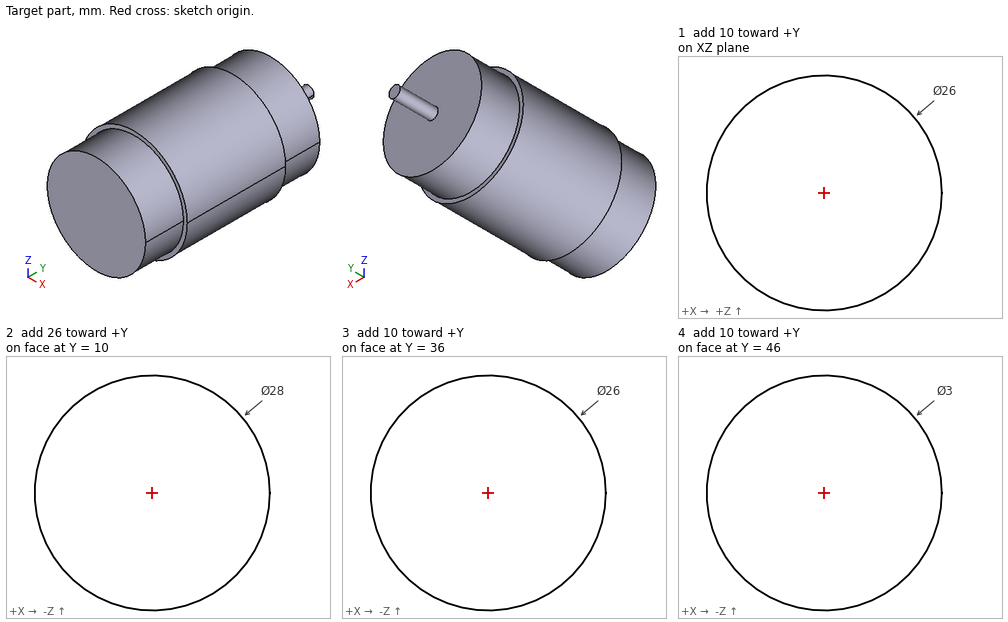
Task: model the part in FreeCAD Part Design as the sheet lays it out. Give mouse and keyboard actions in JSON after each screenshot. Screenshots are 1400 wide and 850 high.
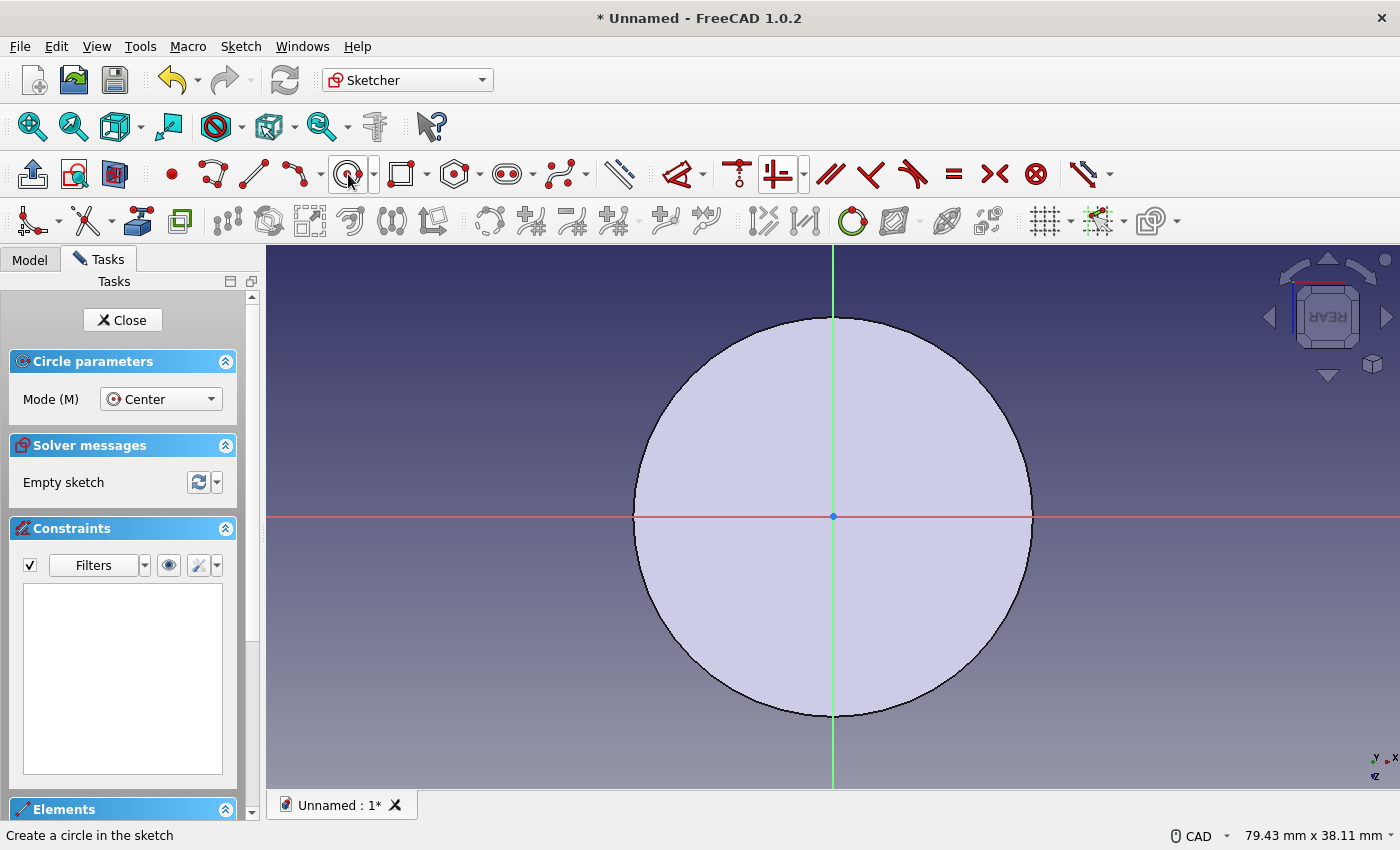
{"action": "left_click", "coordinate": [833, 517]}
{"action": "mouse_move", "coordinate": [964, 386]}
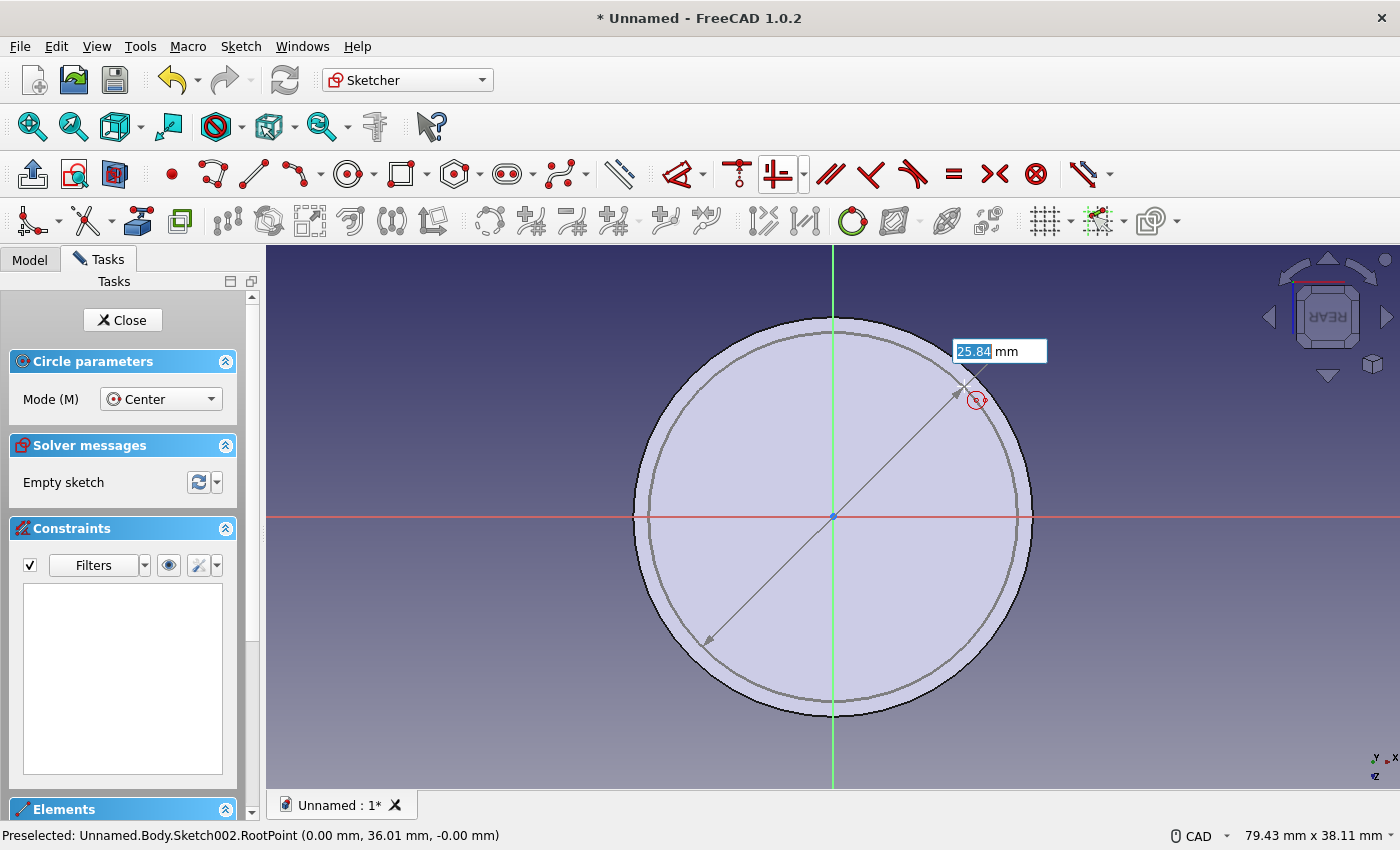
{"action": "type", "text": "26"}
{"action": "key", "text": "Return"}
{"action": "key", "text": "Escape"}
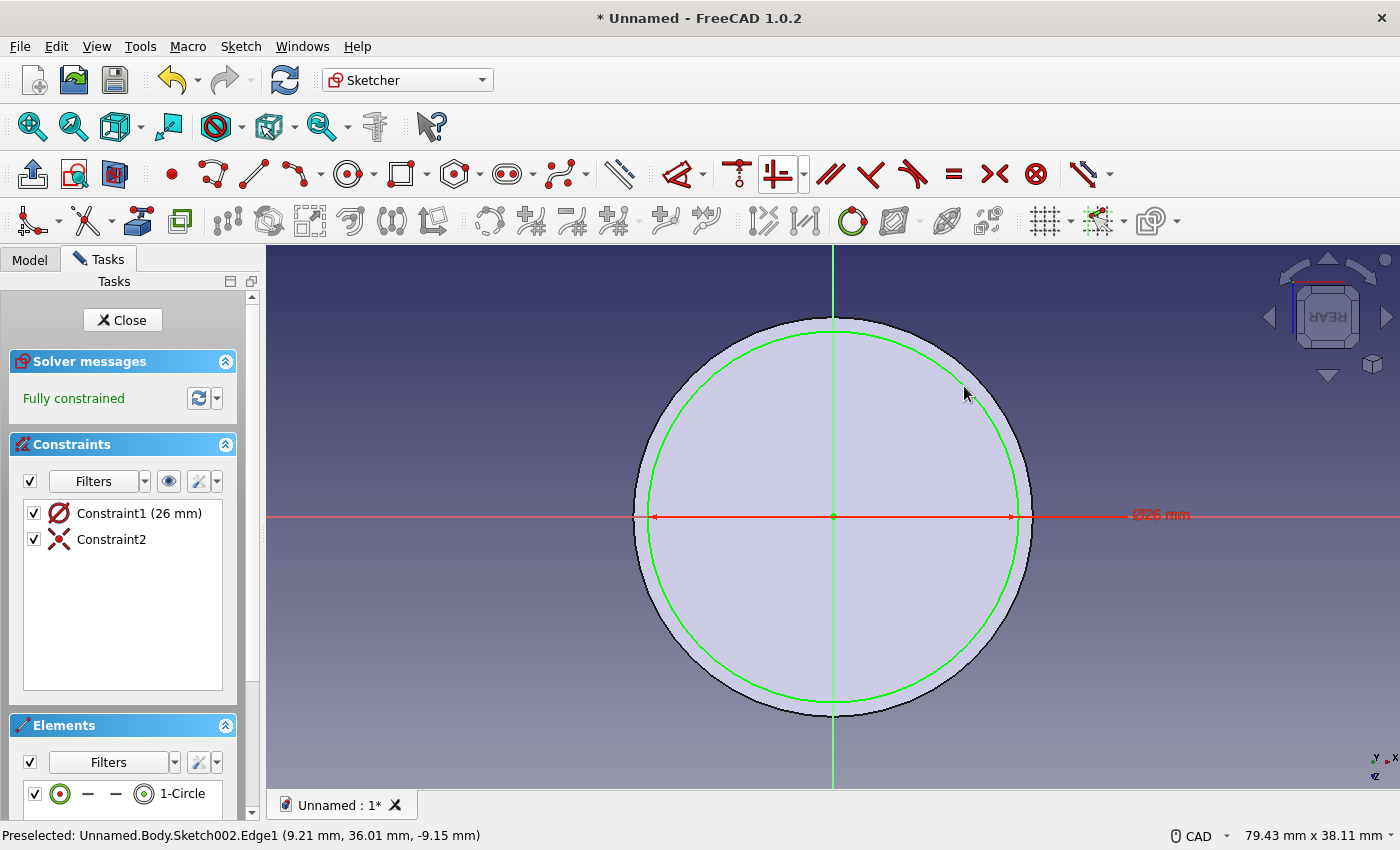
{"action": "left_click", "coordinate": [123, 320]}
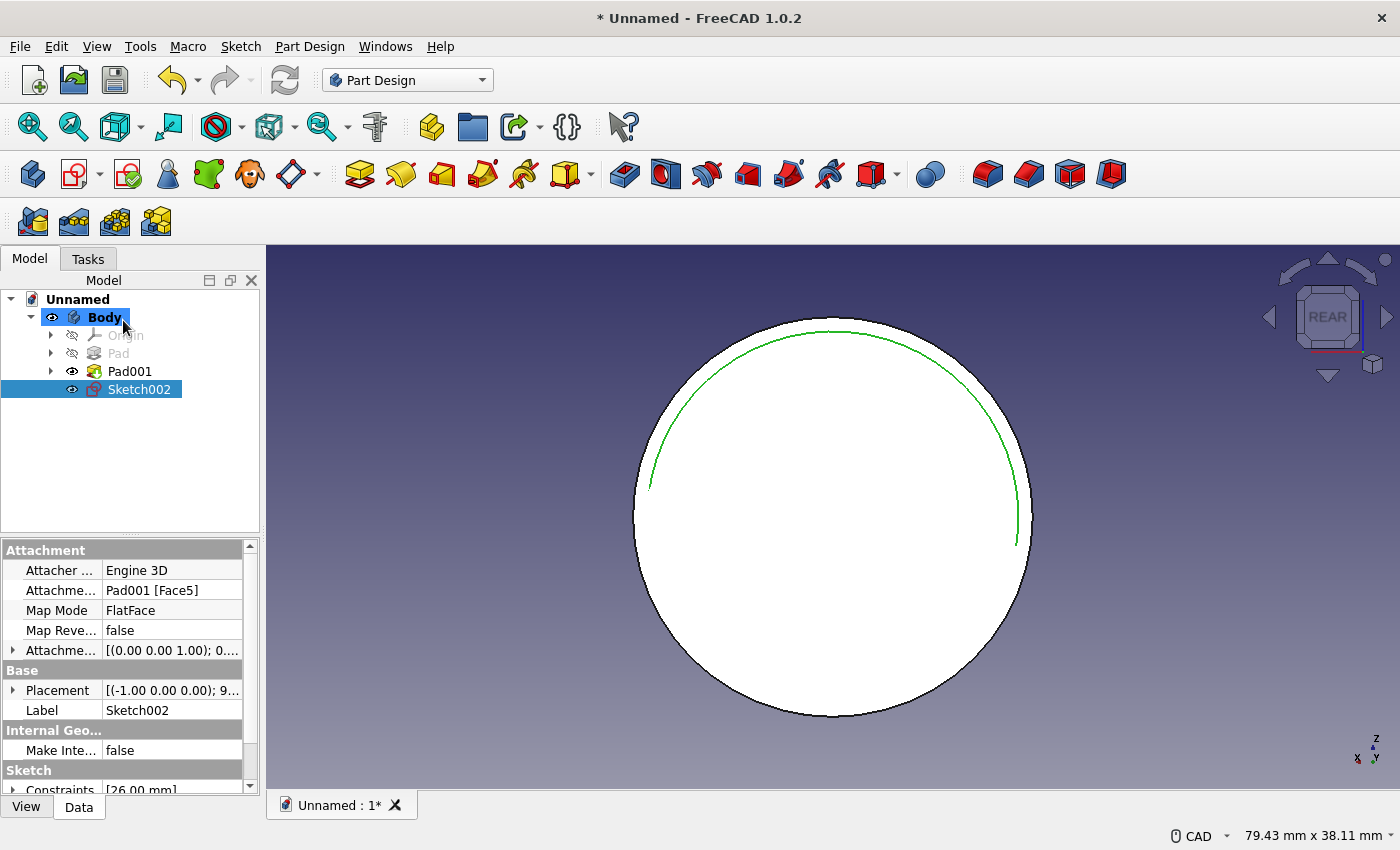
{"action": "left_click", "coordinate": [360, 174]}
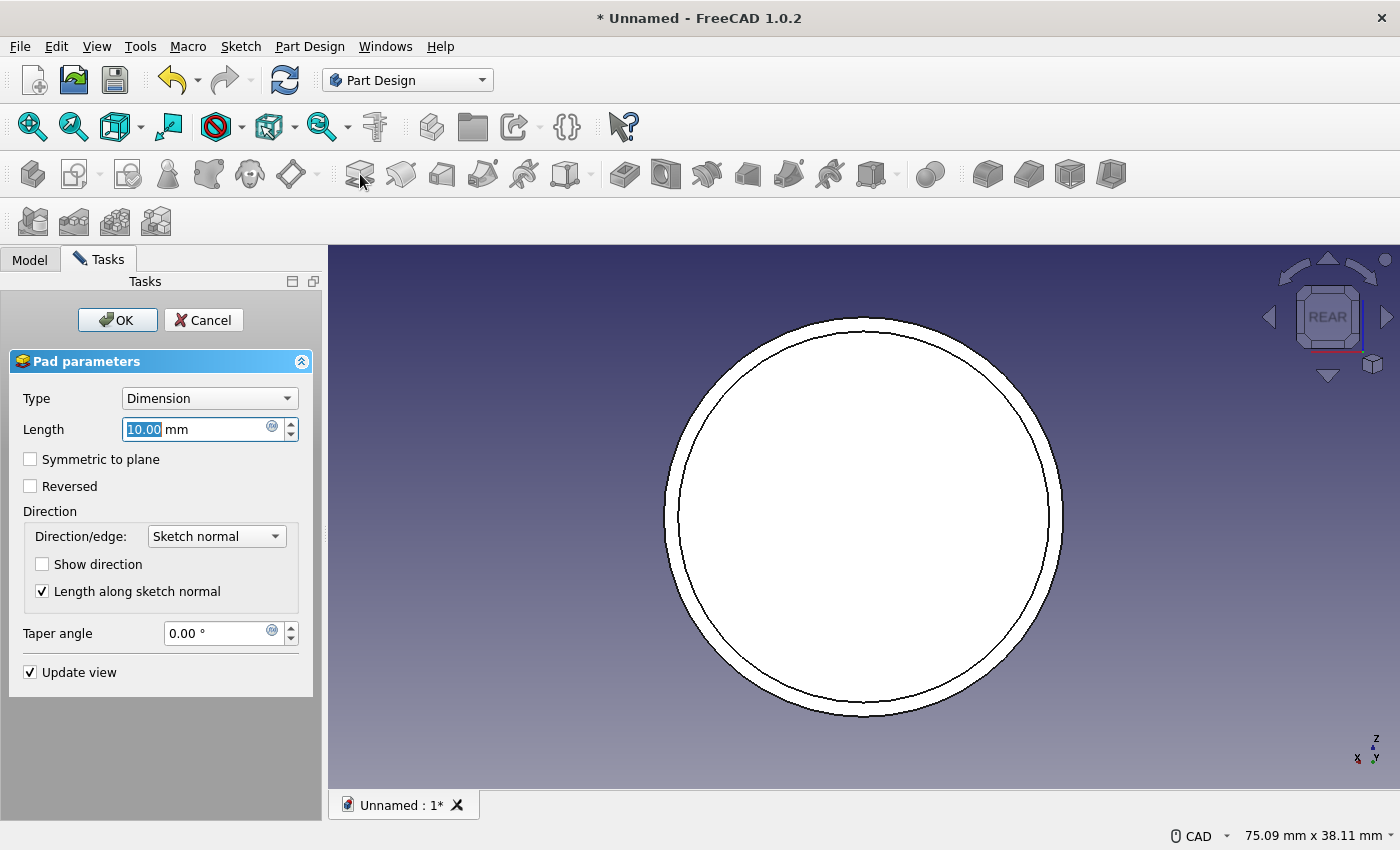
{"action": "type", "text": "10"}
{"action": "key", "text": "Tab"}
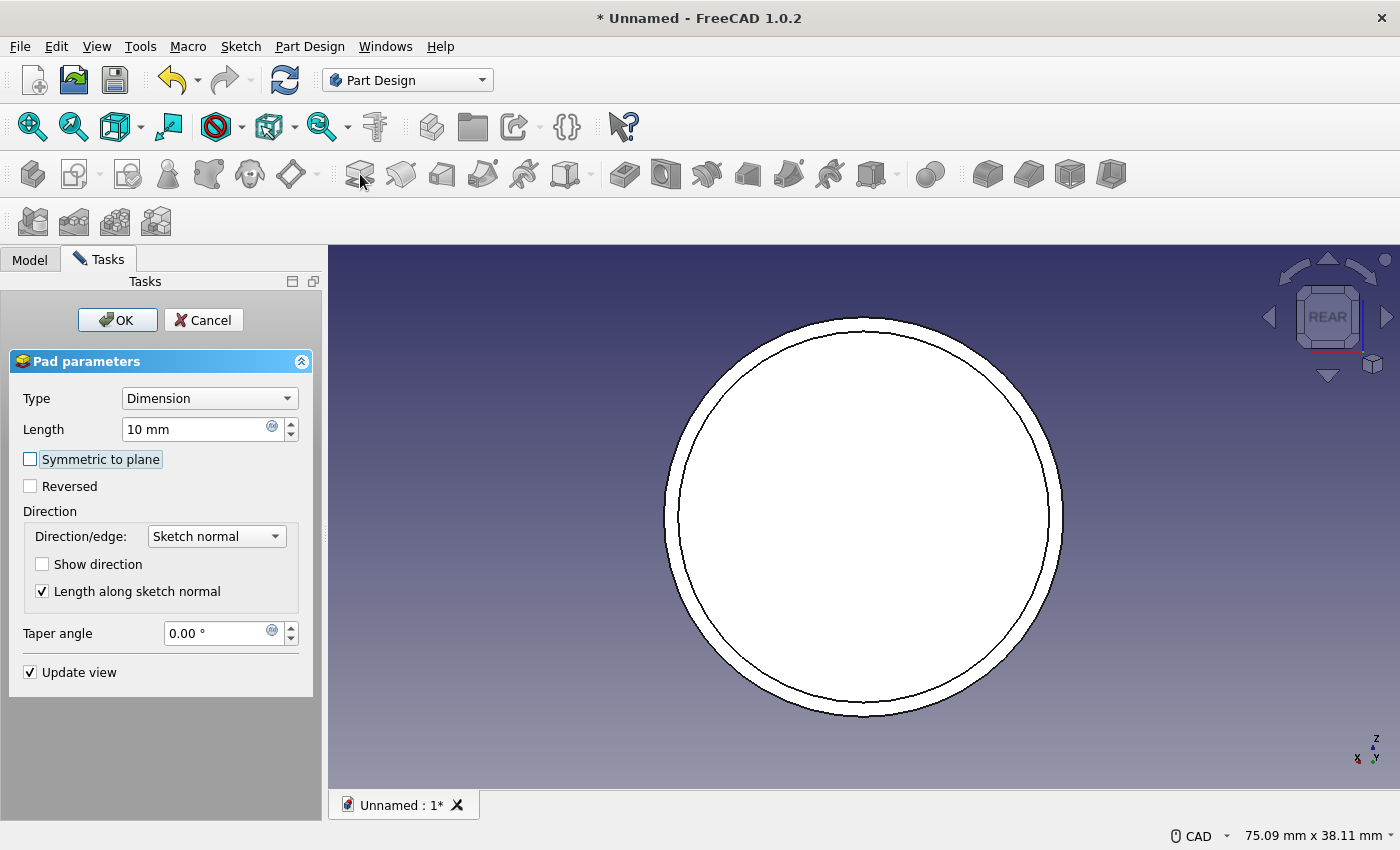
{"action": "left_click", "coordinate": [118, 320]}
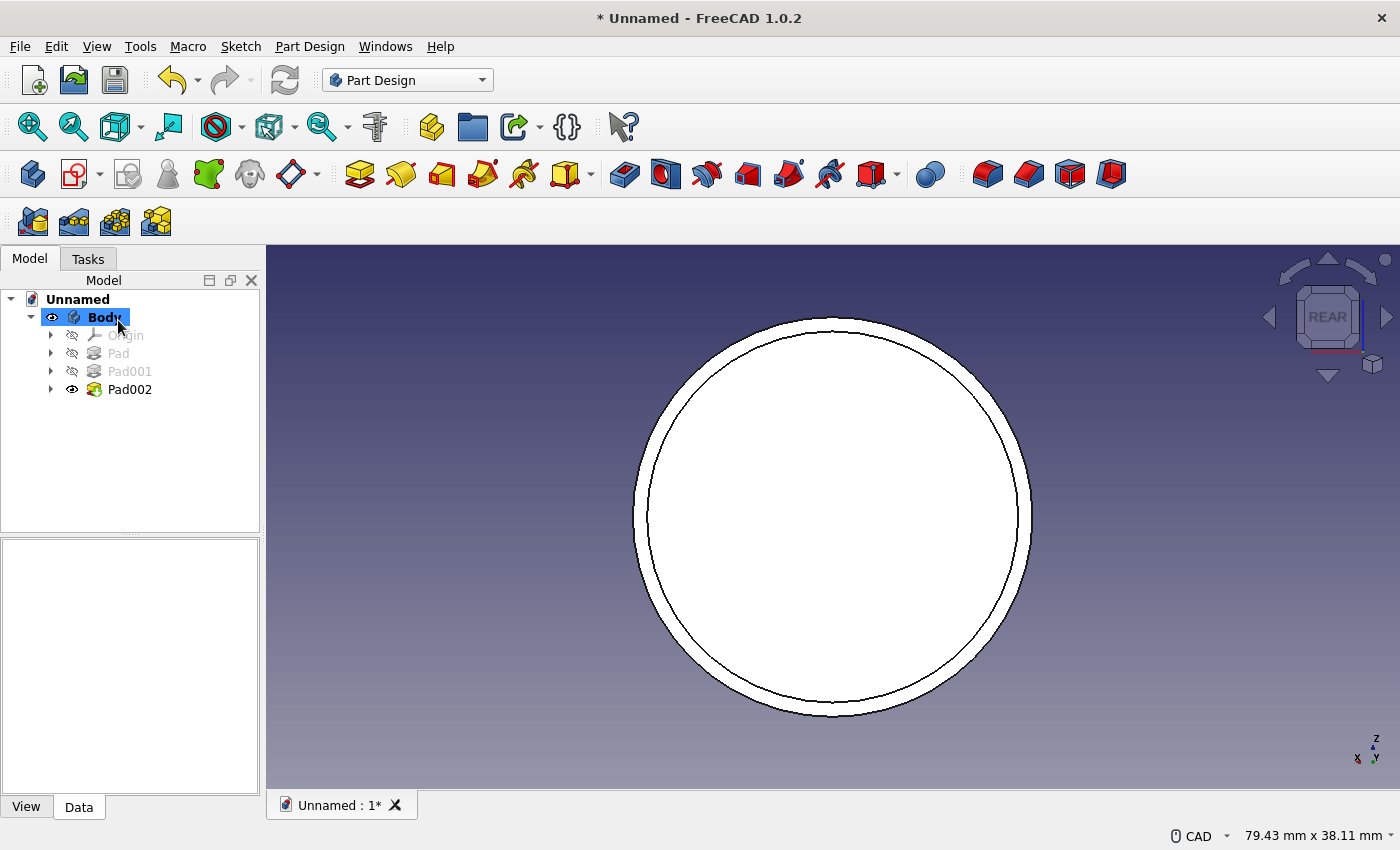
{"action": "left_click", "coordinate": [833, 516]}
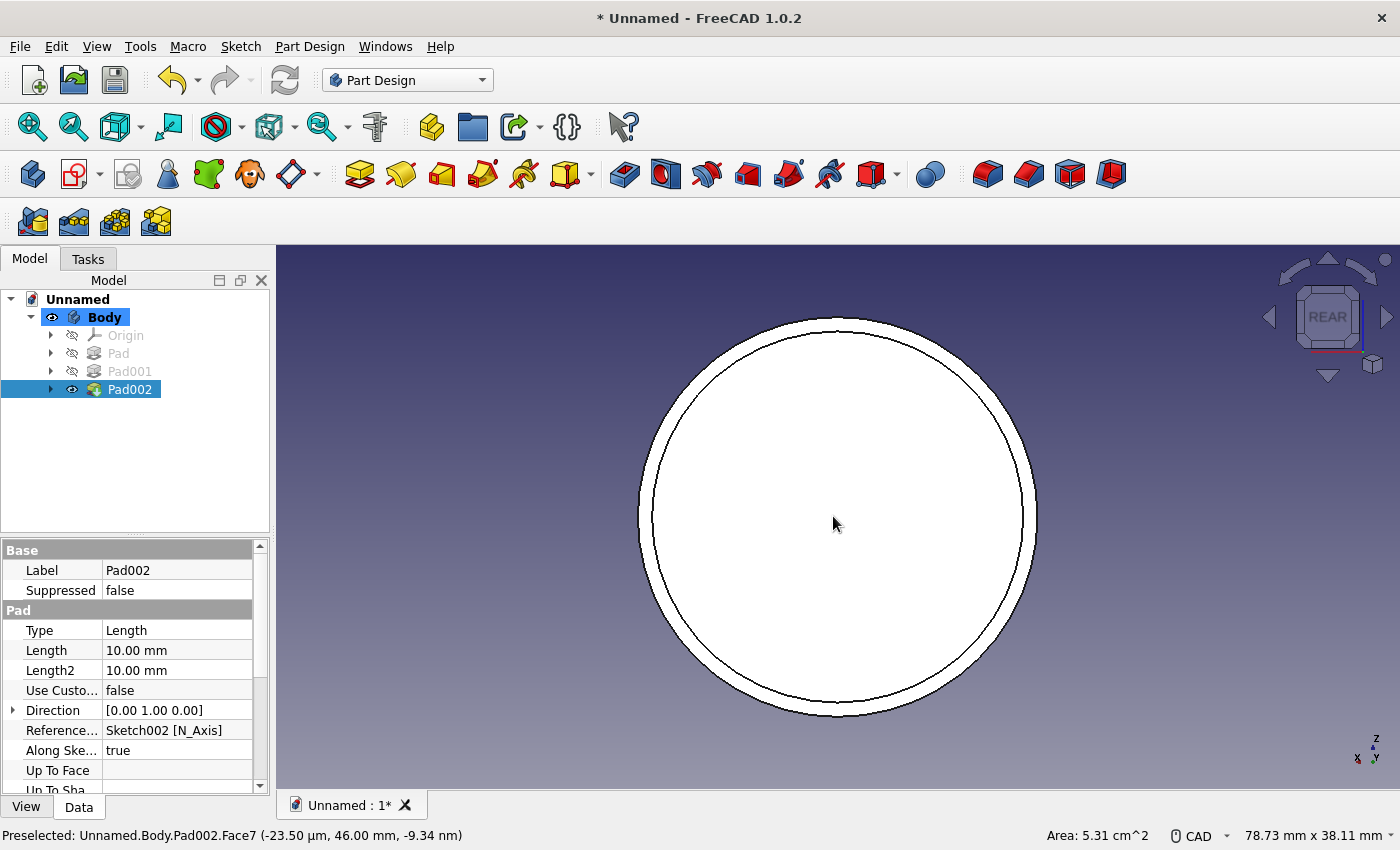
{"action": "left_click", "coordinate": [74, 174]}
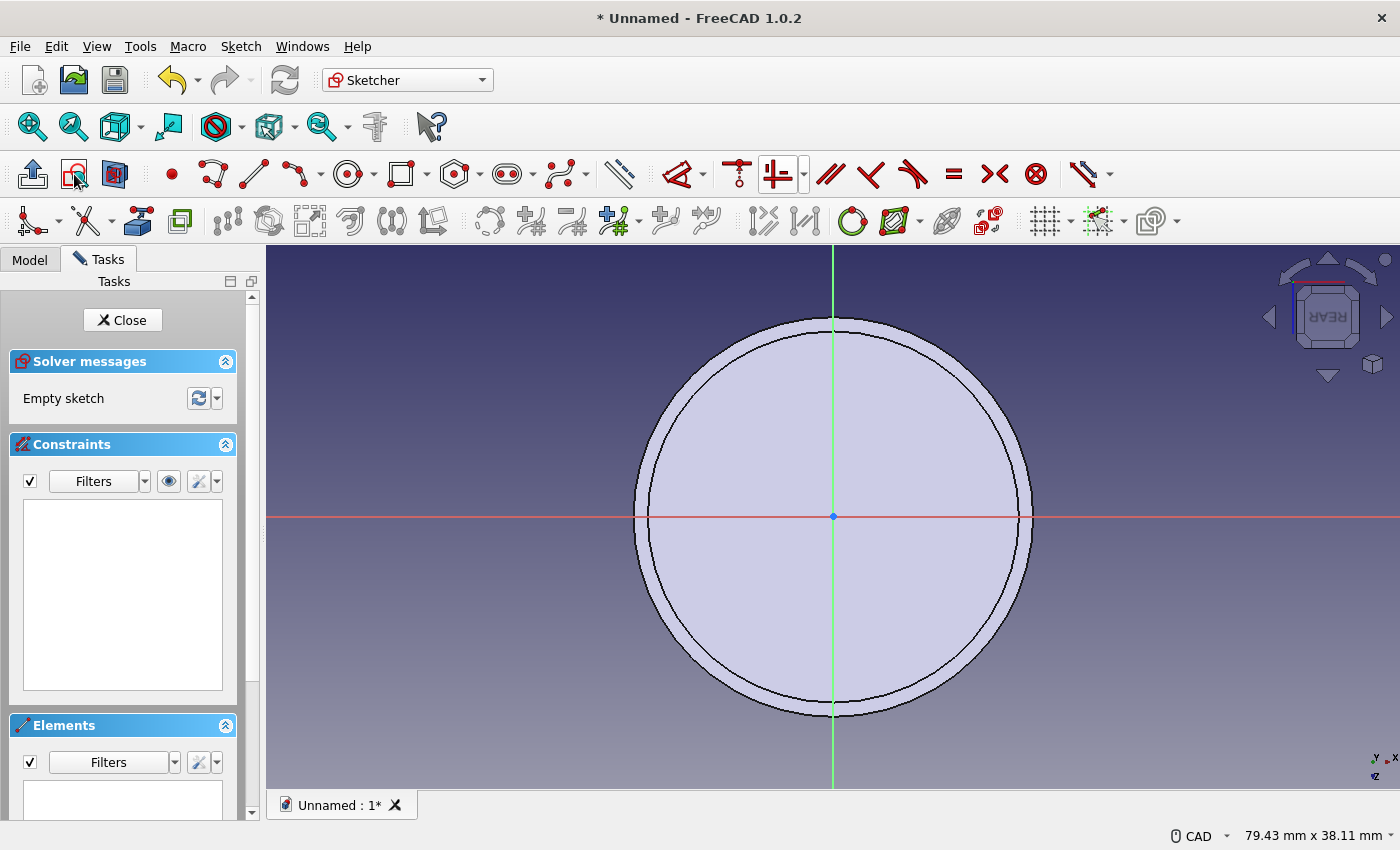
{"action": "scroll", "coordinate": [844, 517], "scroll_direction": "up", "scroll_amount": 10}